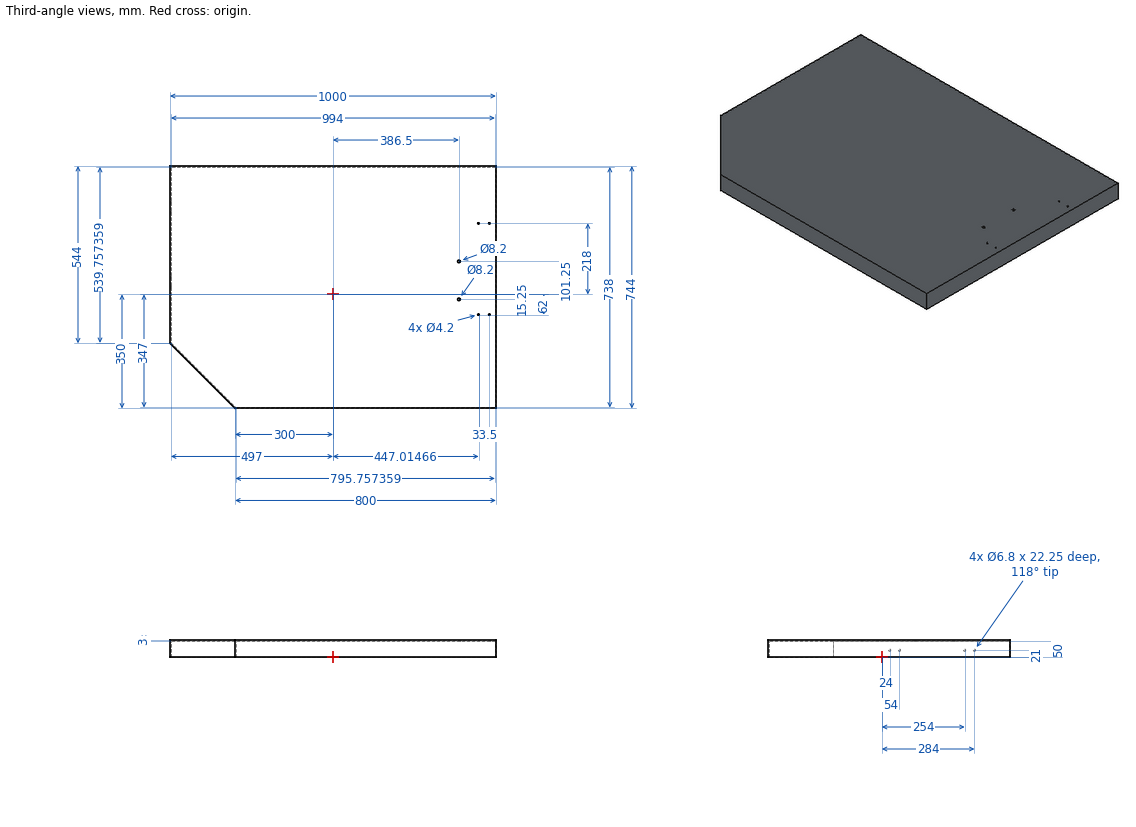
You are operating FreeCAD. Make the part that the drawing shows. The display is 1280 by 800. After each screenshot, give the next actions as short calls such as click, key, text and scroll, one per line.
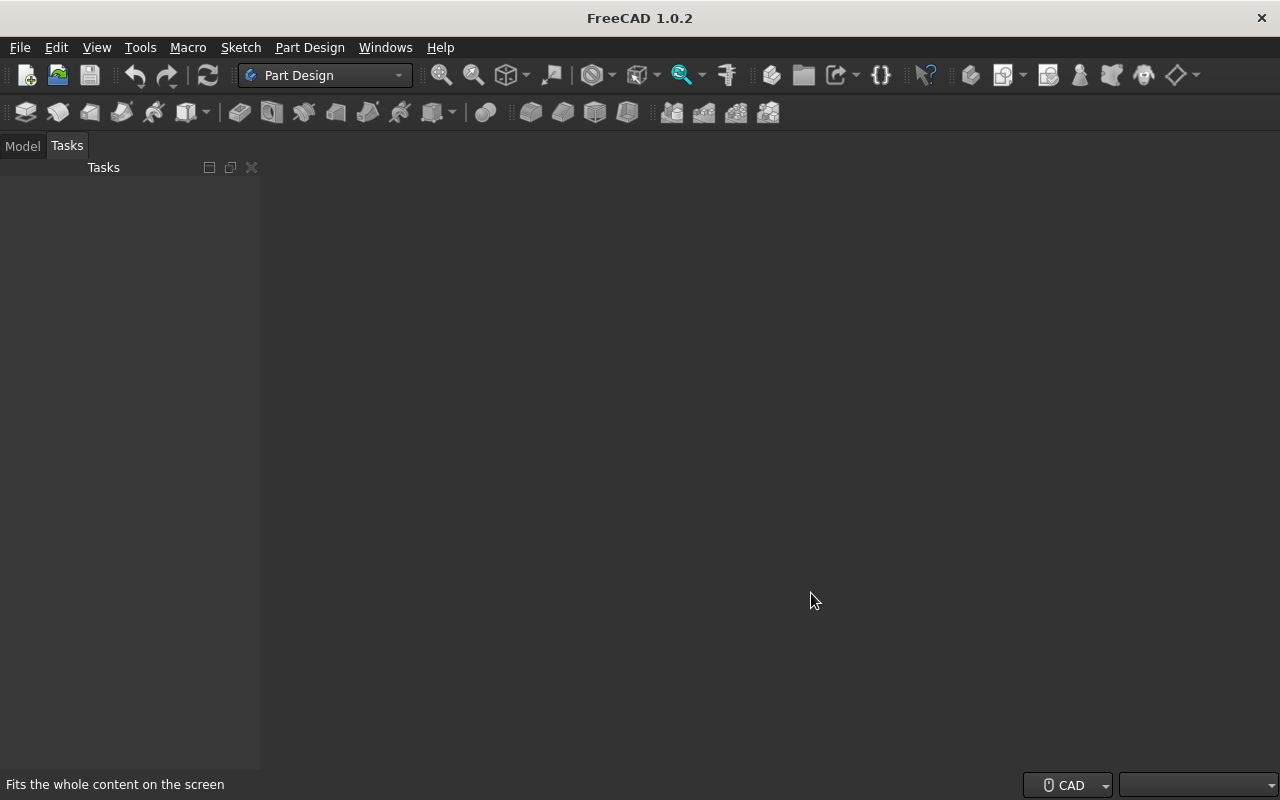
click(26, 76)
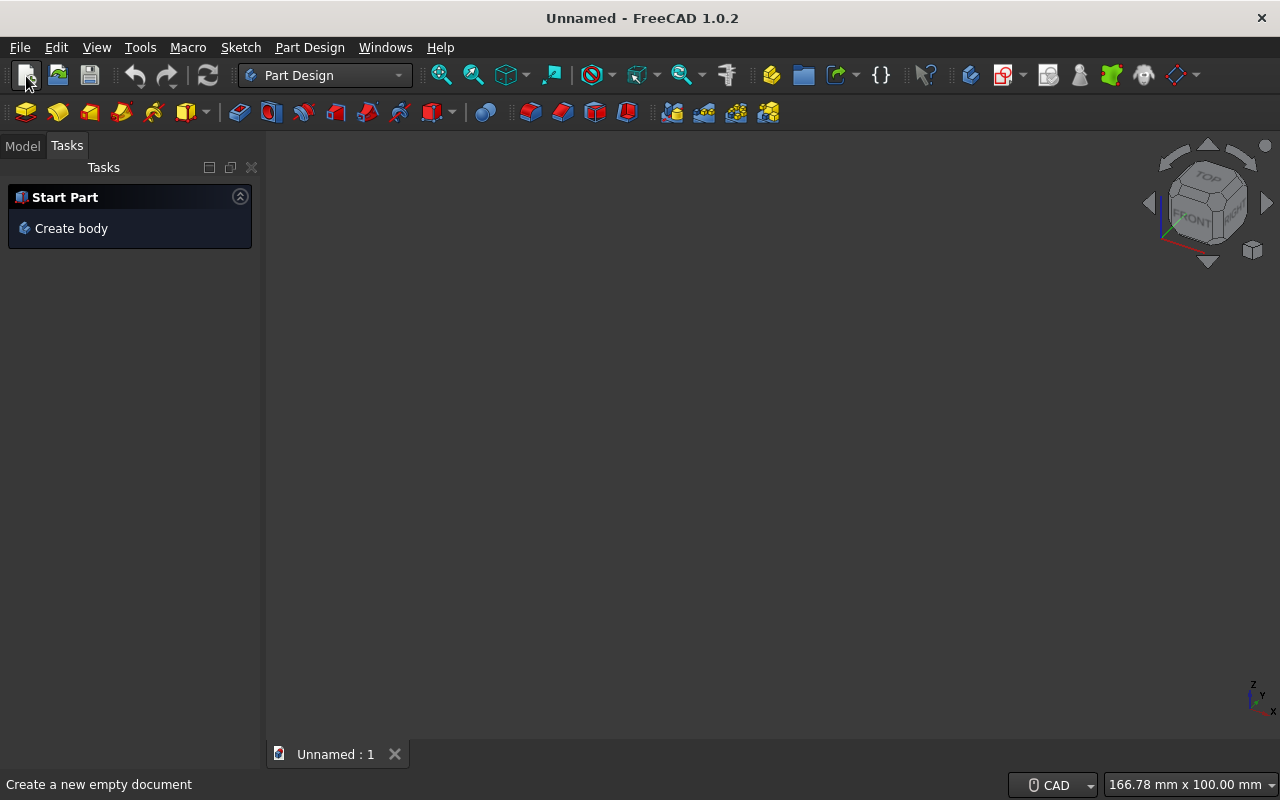
click(1004, 76)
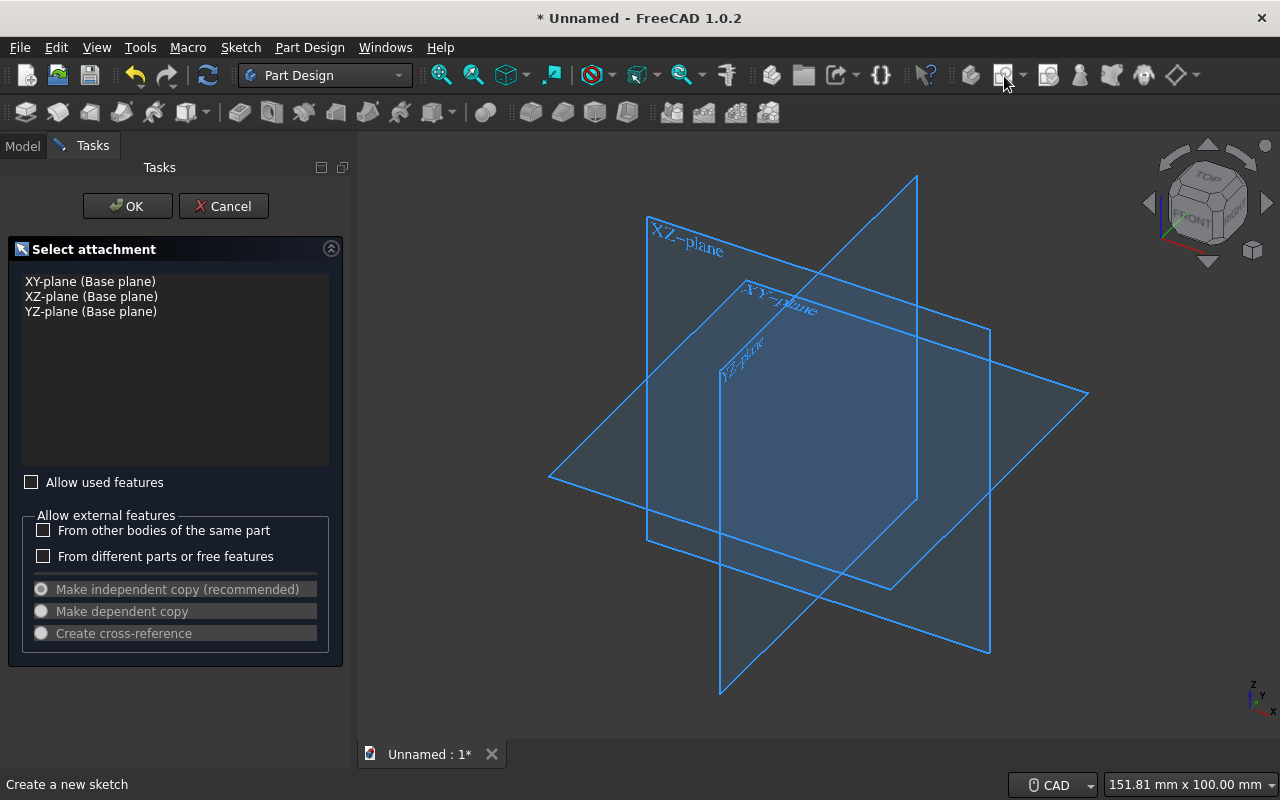
click(82, 282)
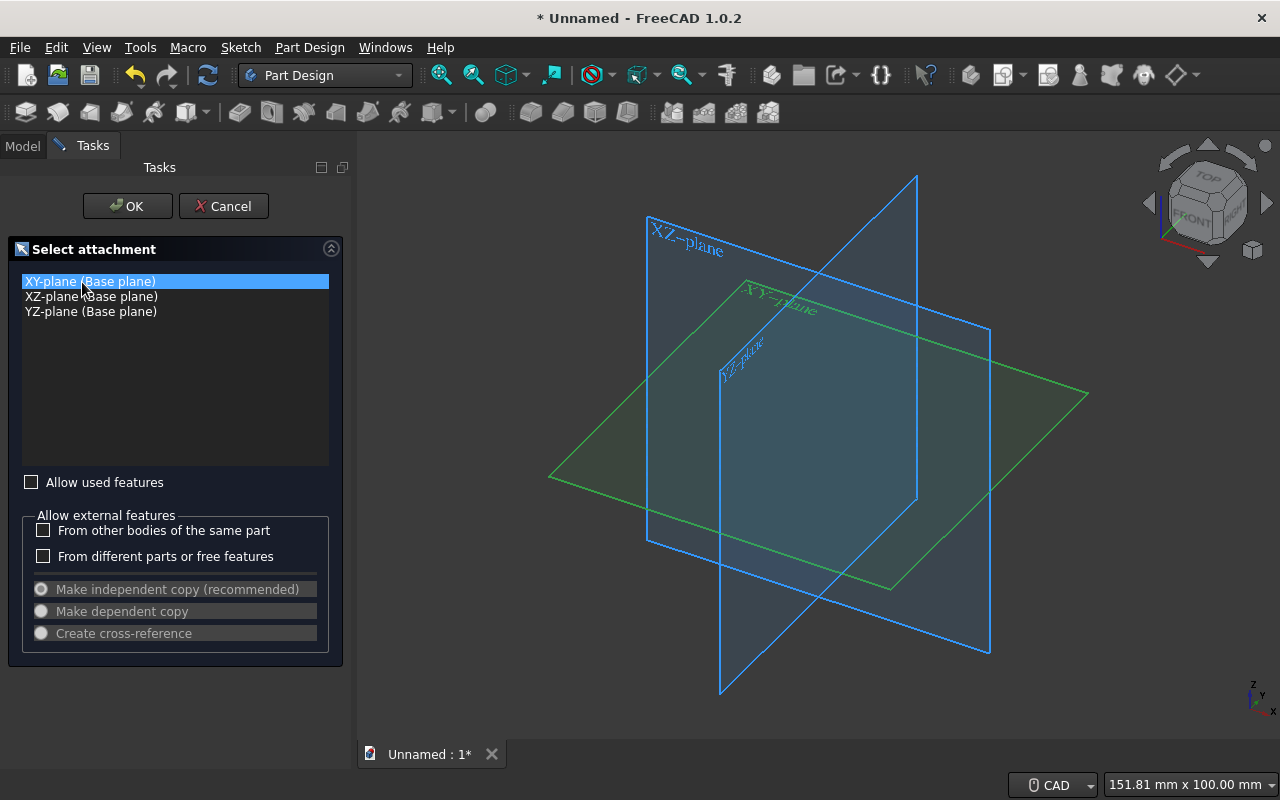
click(128, 206)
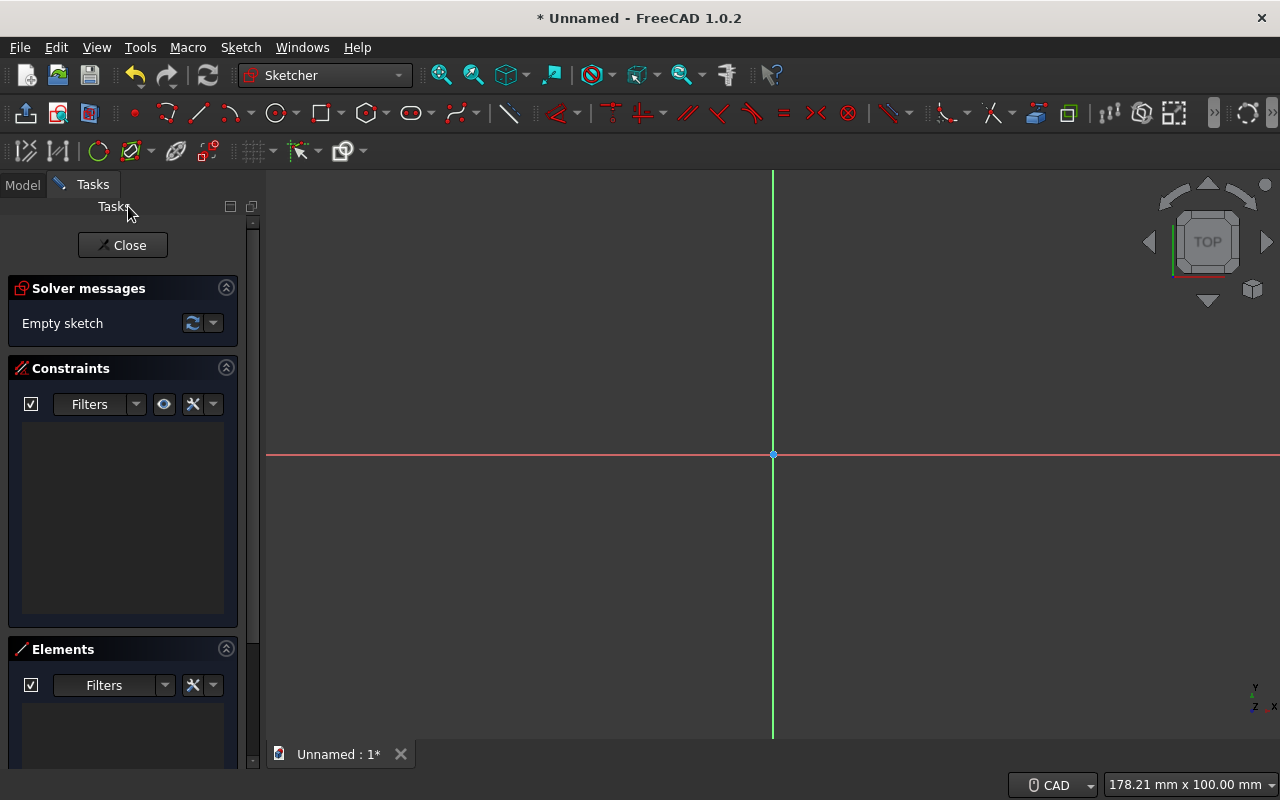
scroll(698, 467, down, 12)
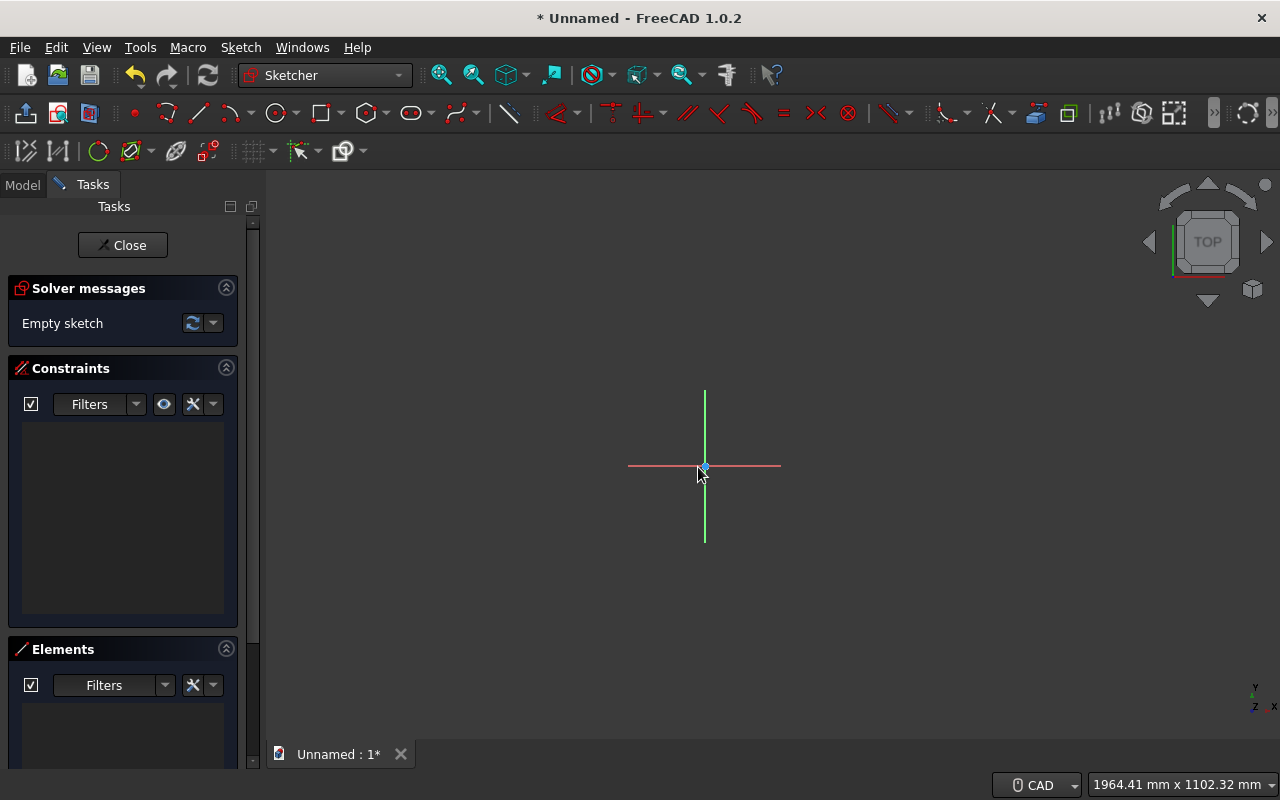
click(168, 114)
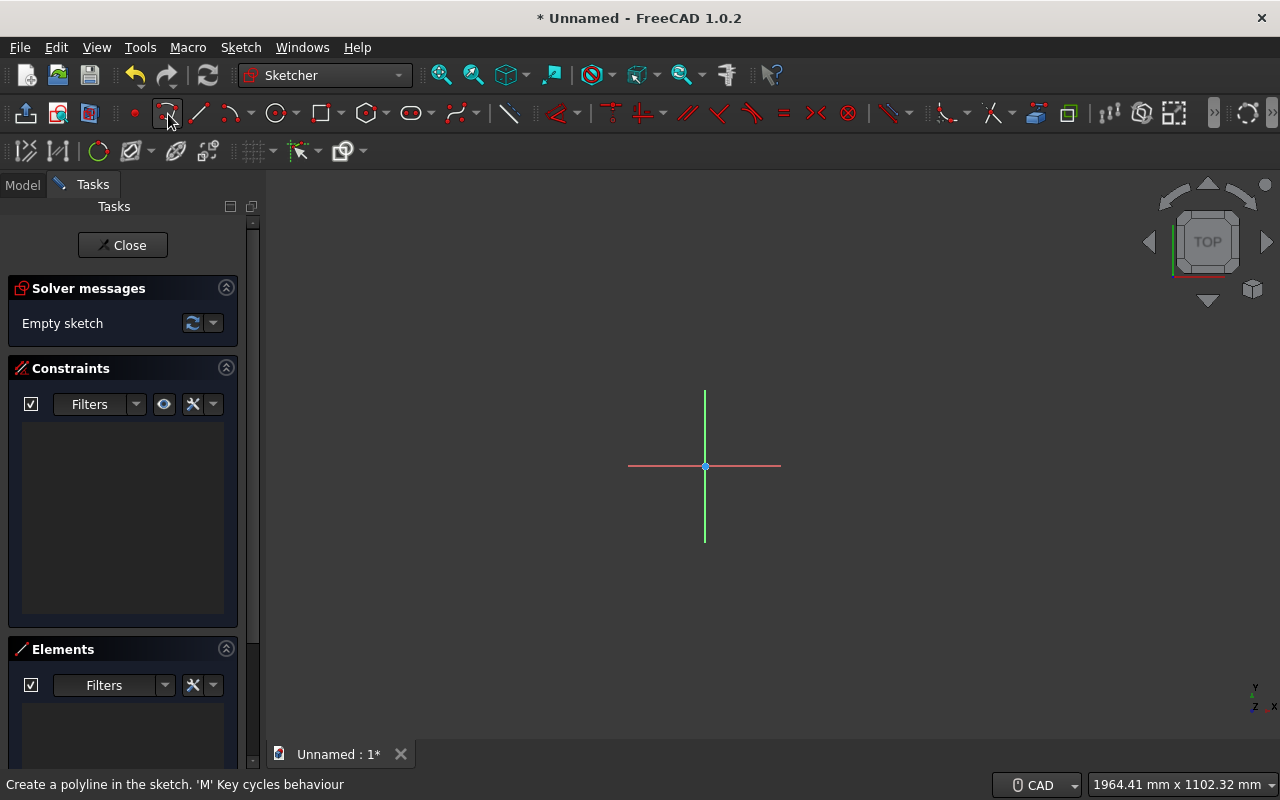
click(550, 647)
click(963, 647)
click(963, 263)
click(447, 263)
click(447, 544)
click(550, 648)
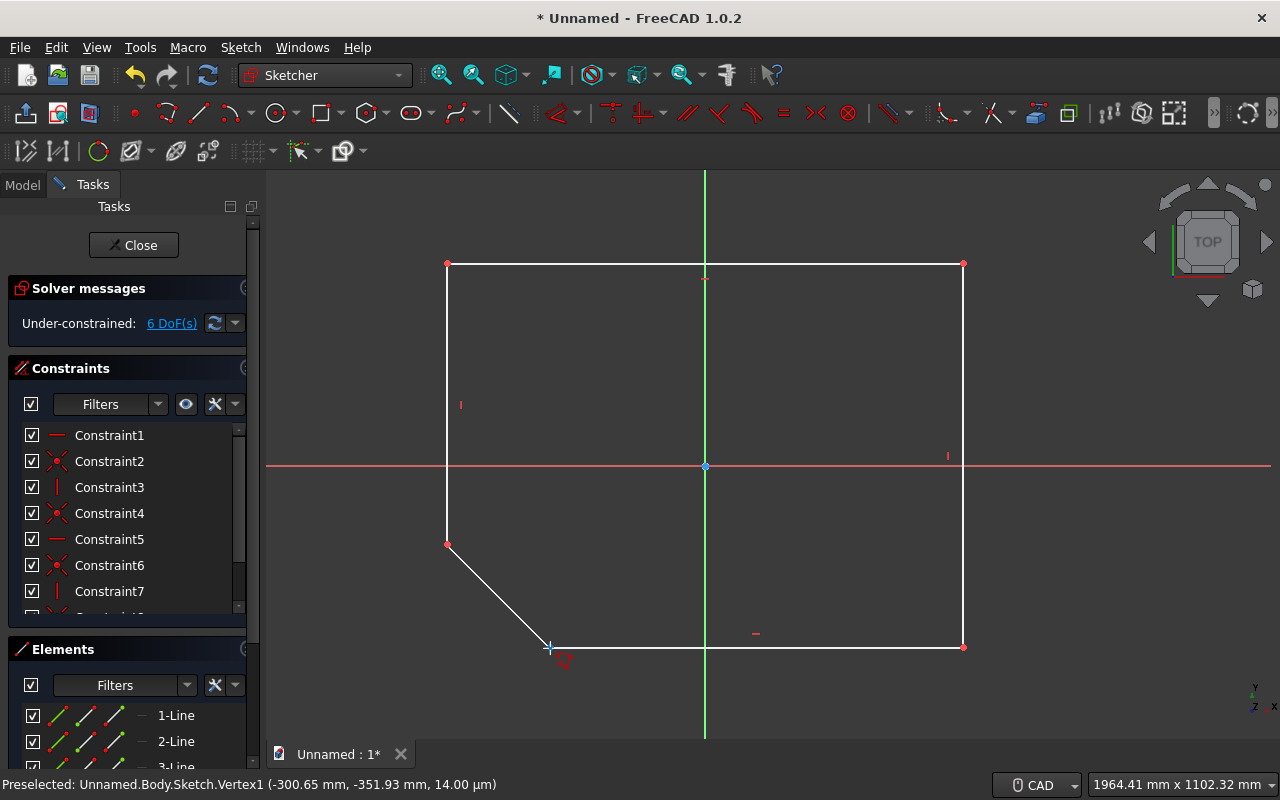
scroll(551, 645, up, 12)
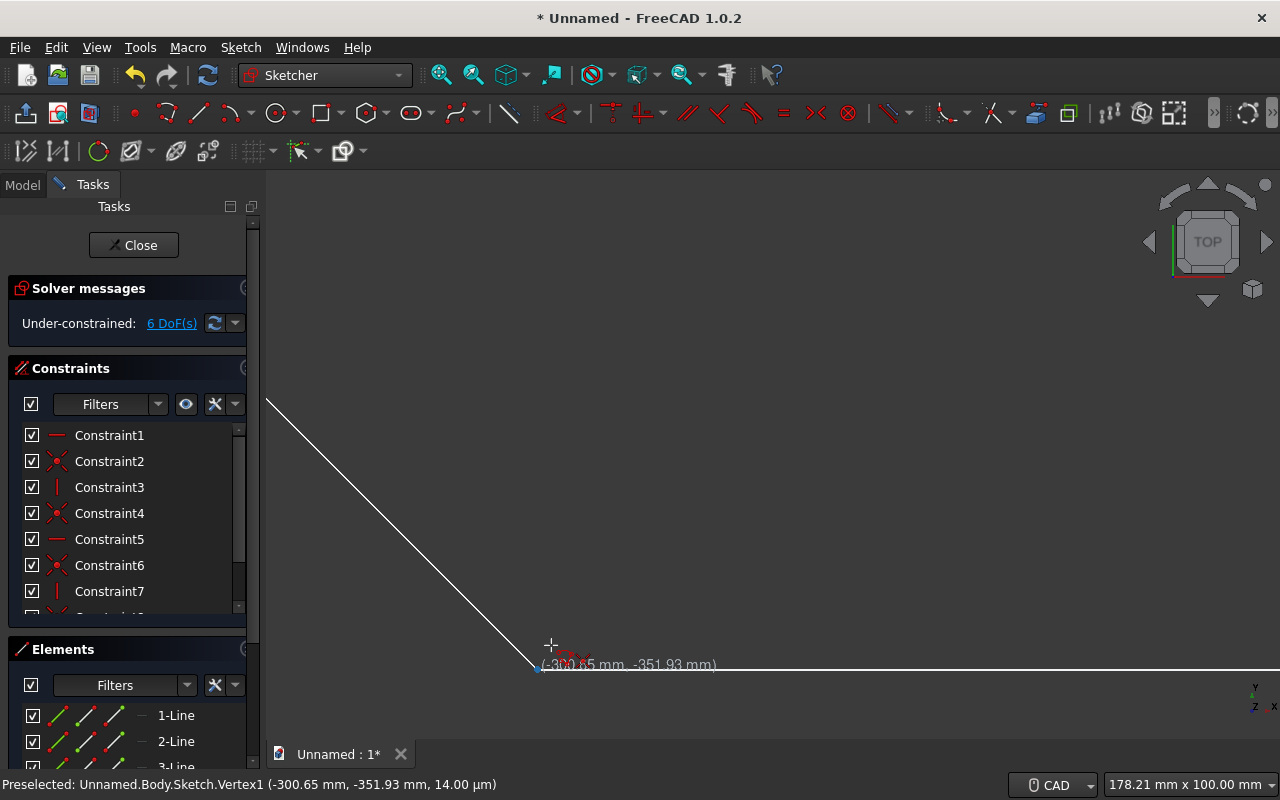
click(548, 642)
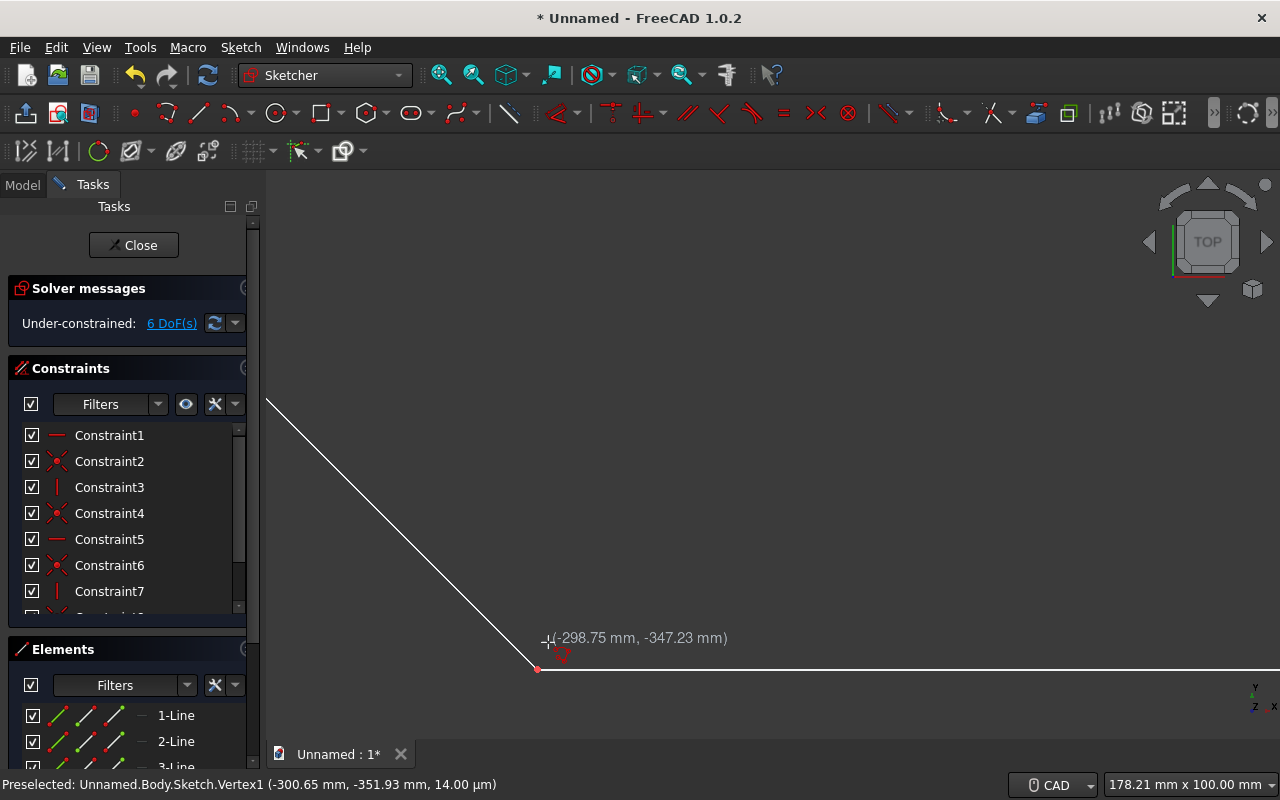
scroll(551, 645, down, 12)